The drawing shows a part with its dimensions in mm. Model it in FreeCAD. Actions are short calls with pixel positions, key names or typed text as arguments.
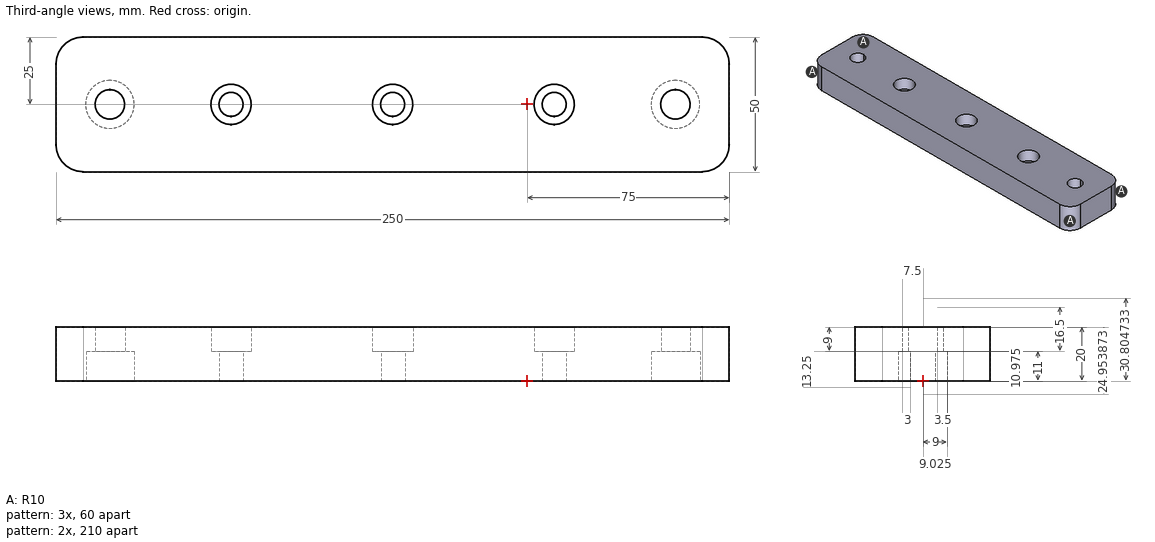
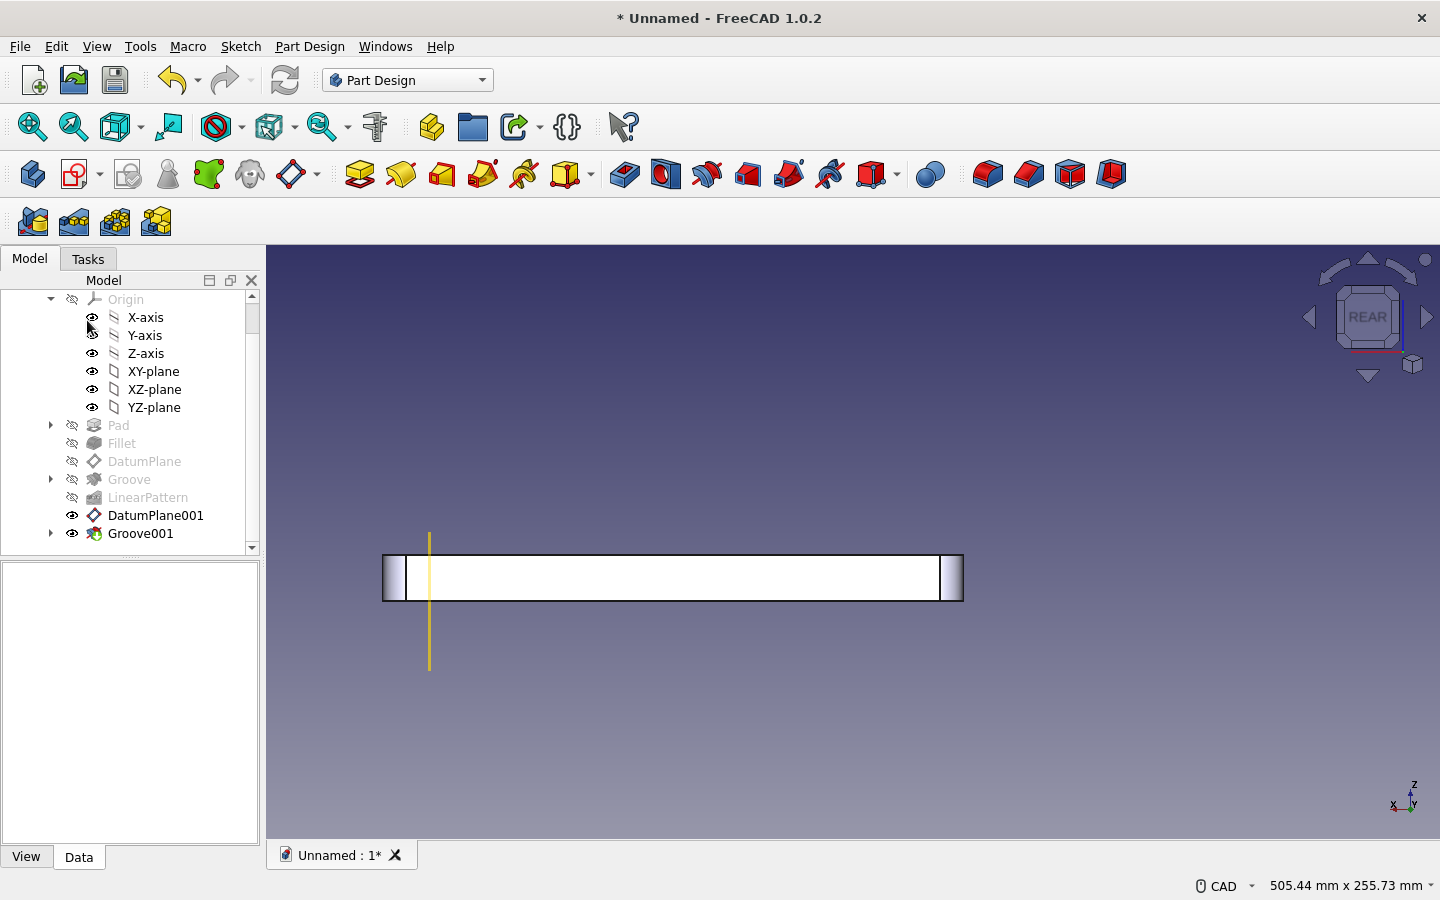
click(117, 515)
key(space)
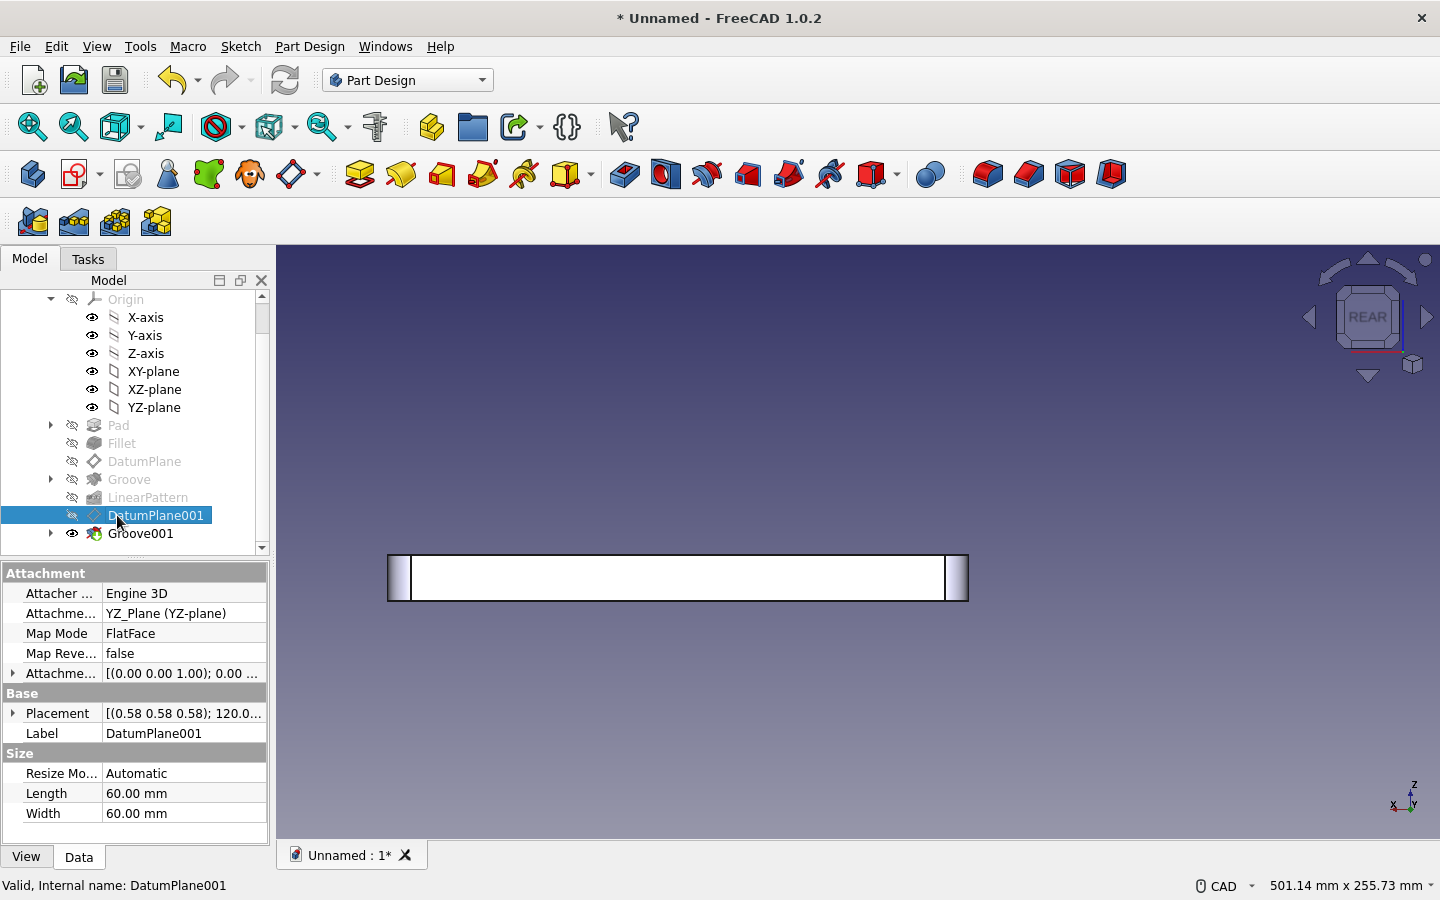
click(117, 533)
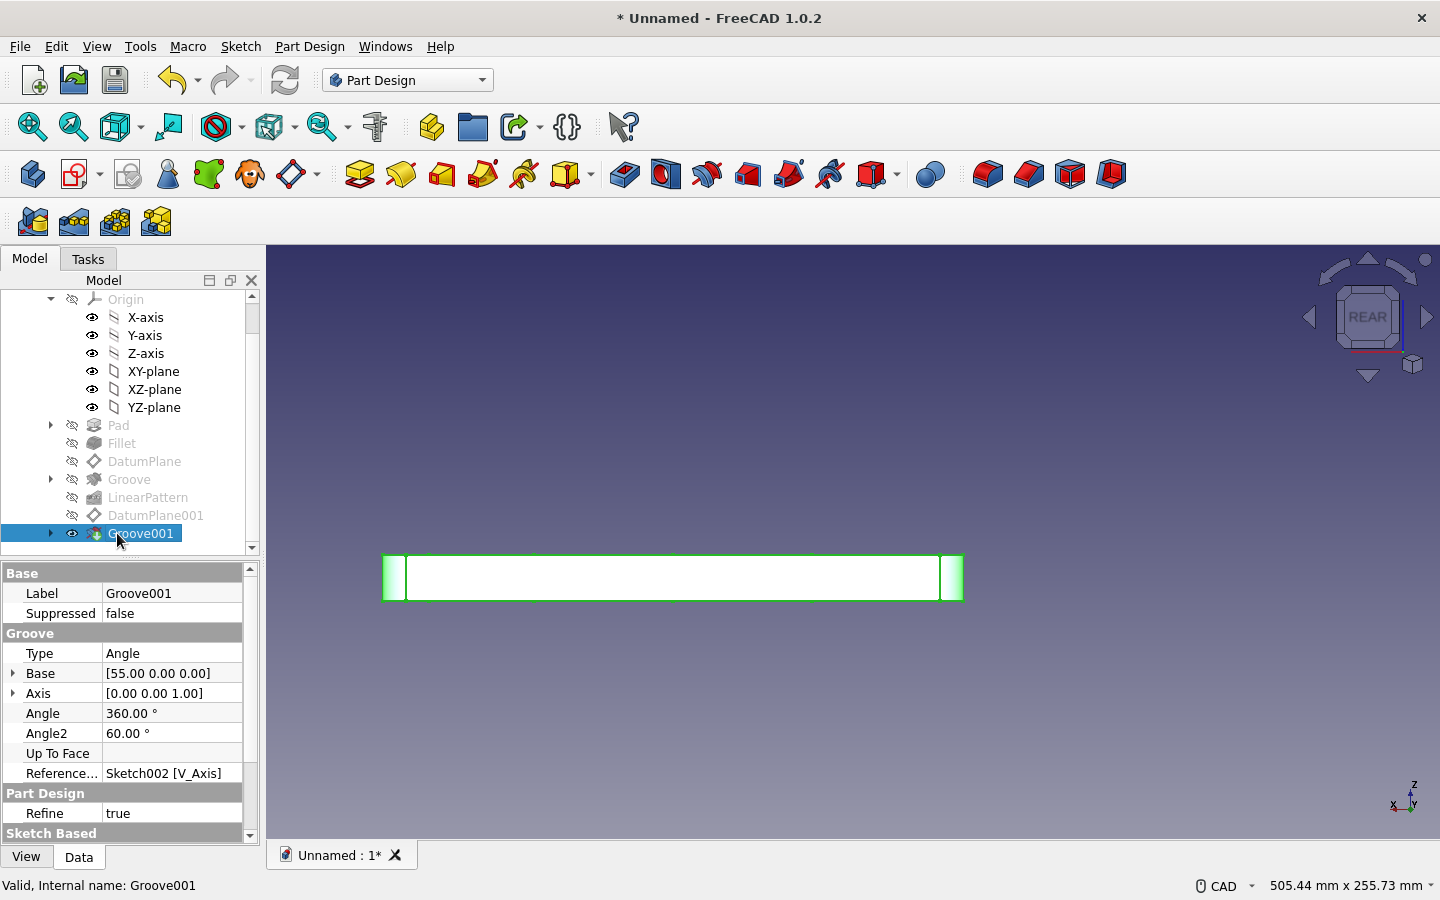
click(74, 222)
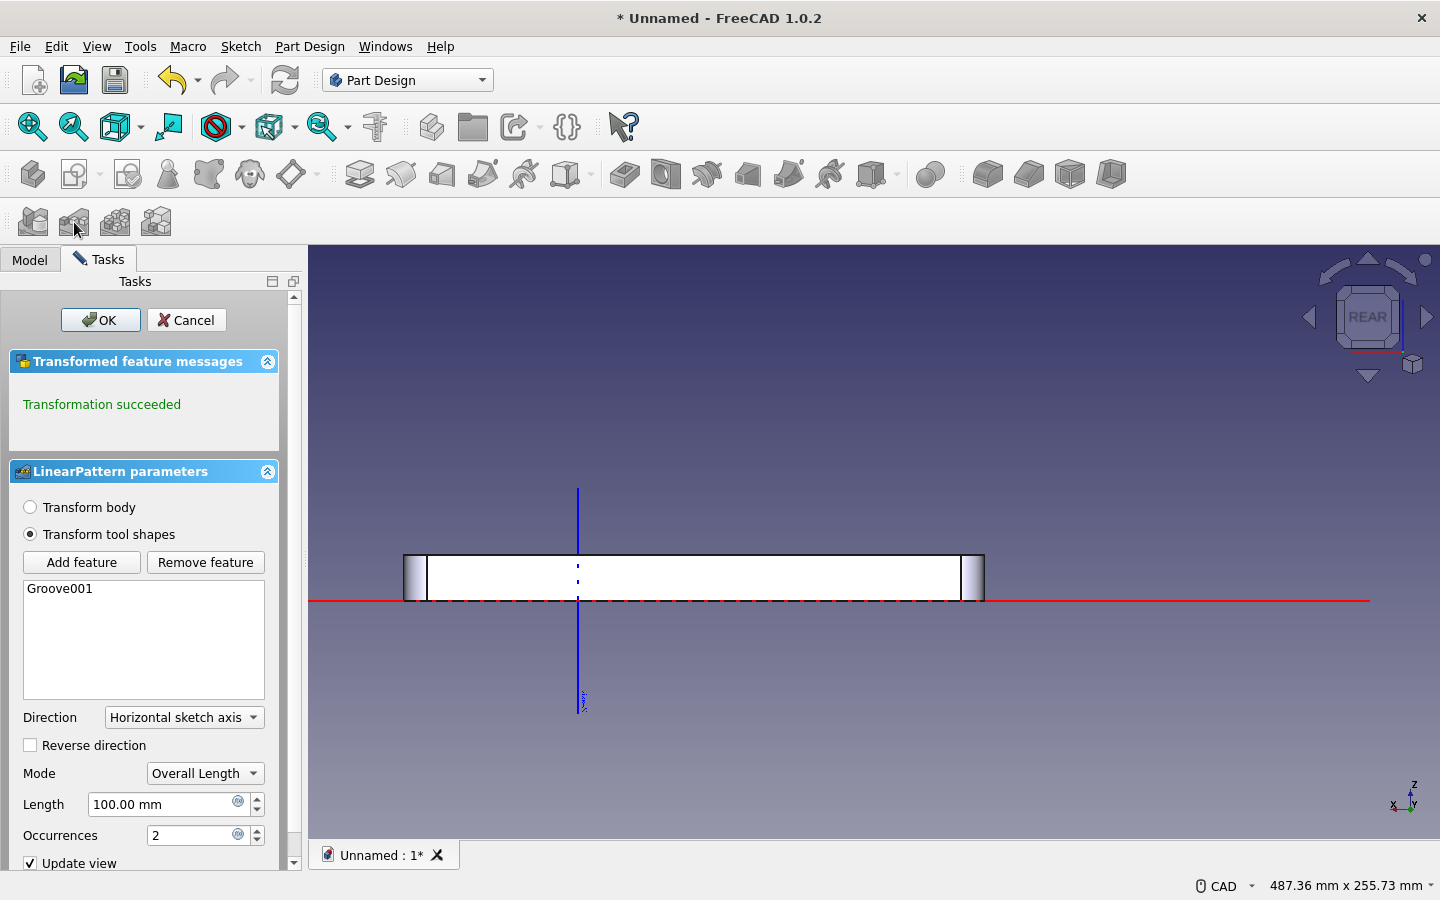
click(185, 718)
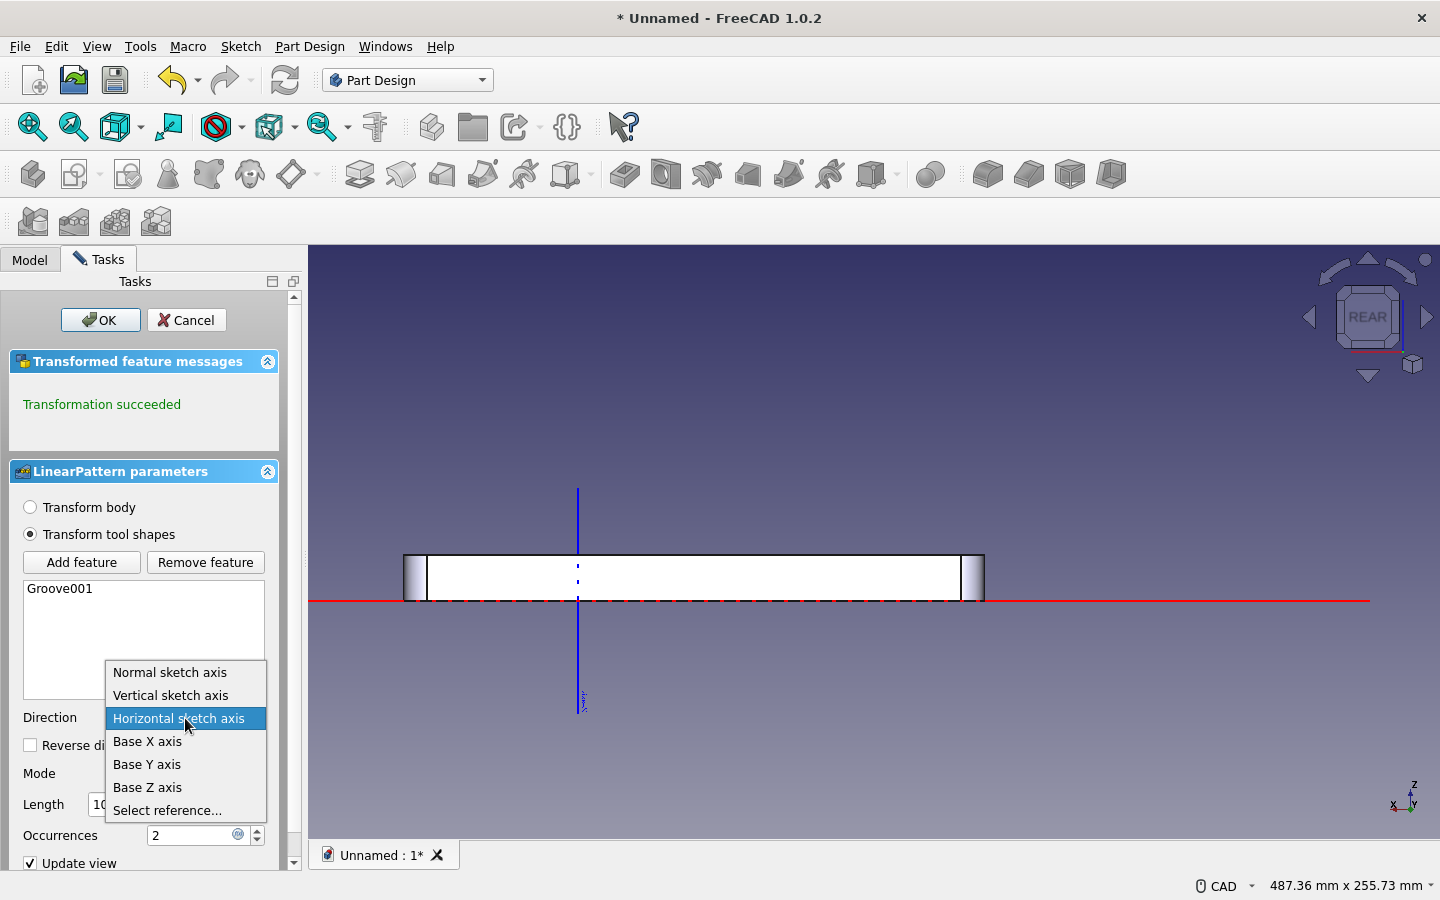
click(184, 742)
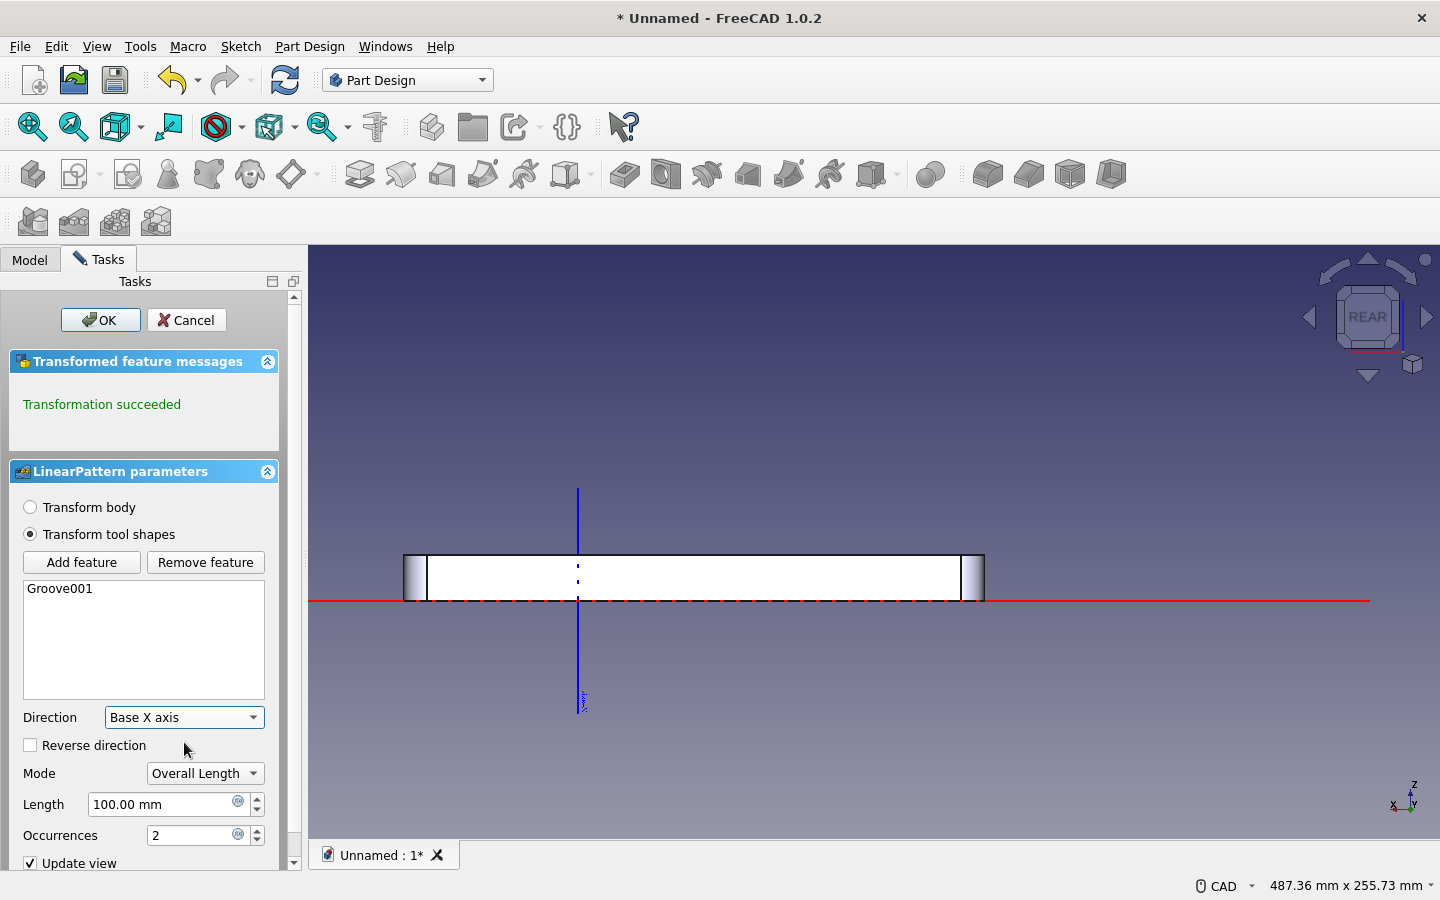
click(206, 774)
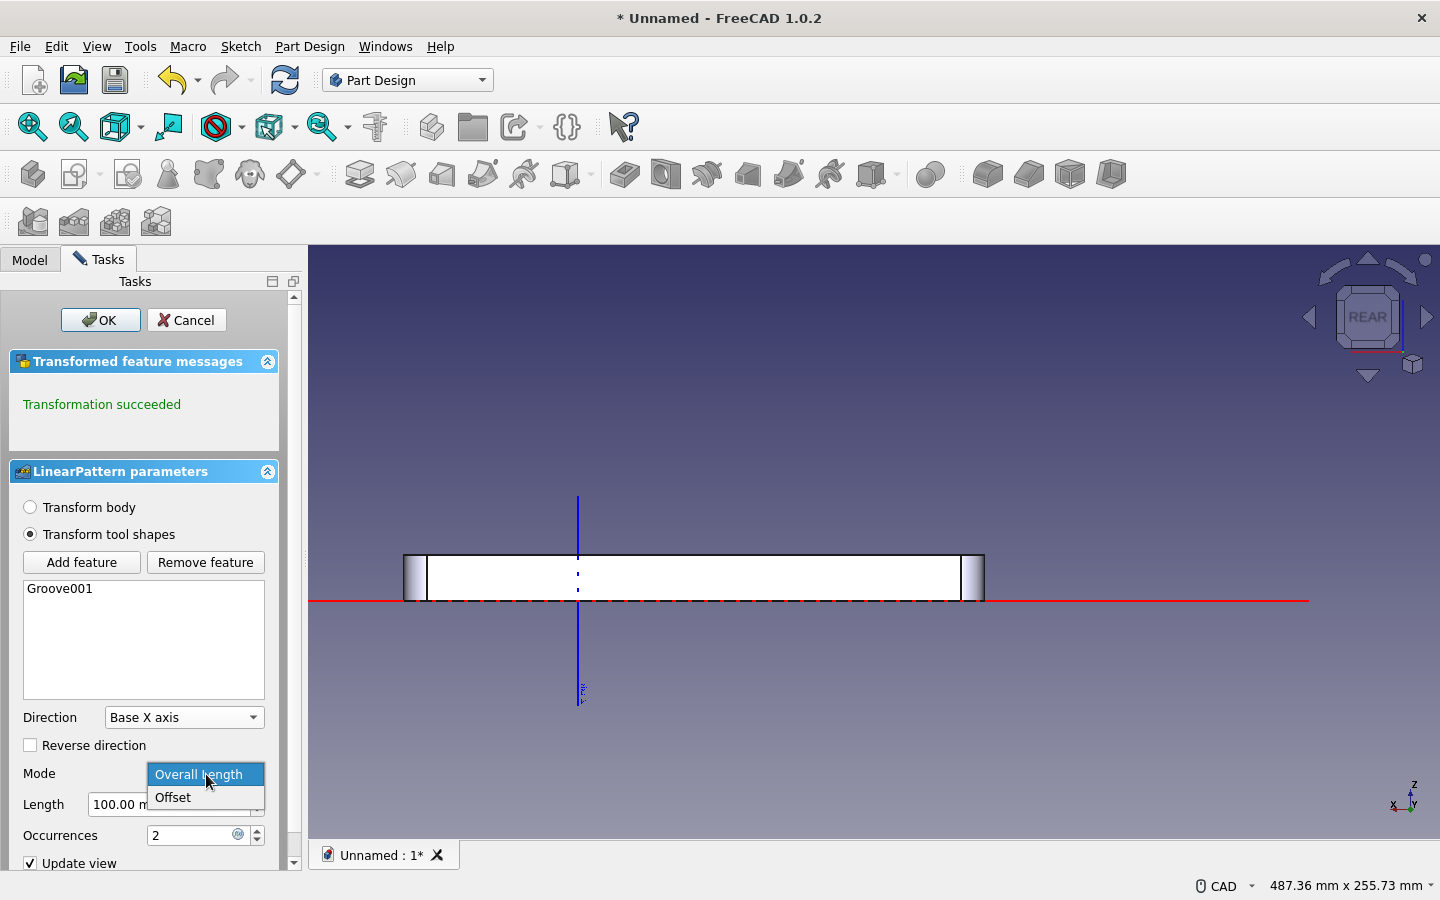
click(204, 798)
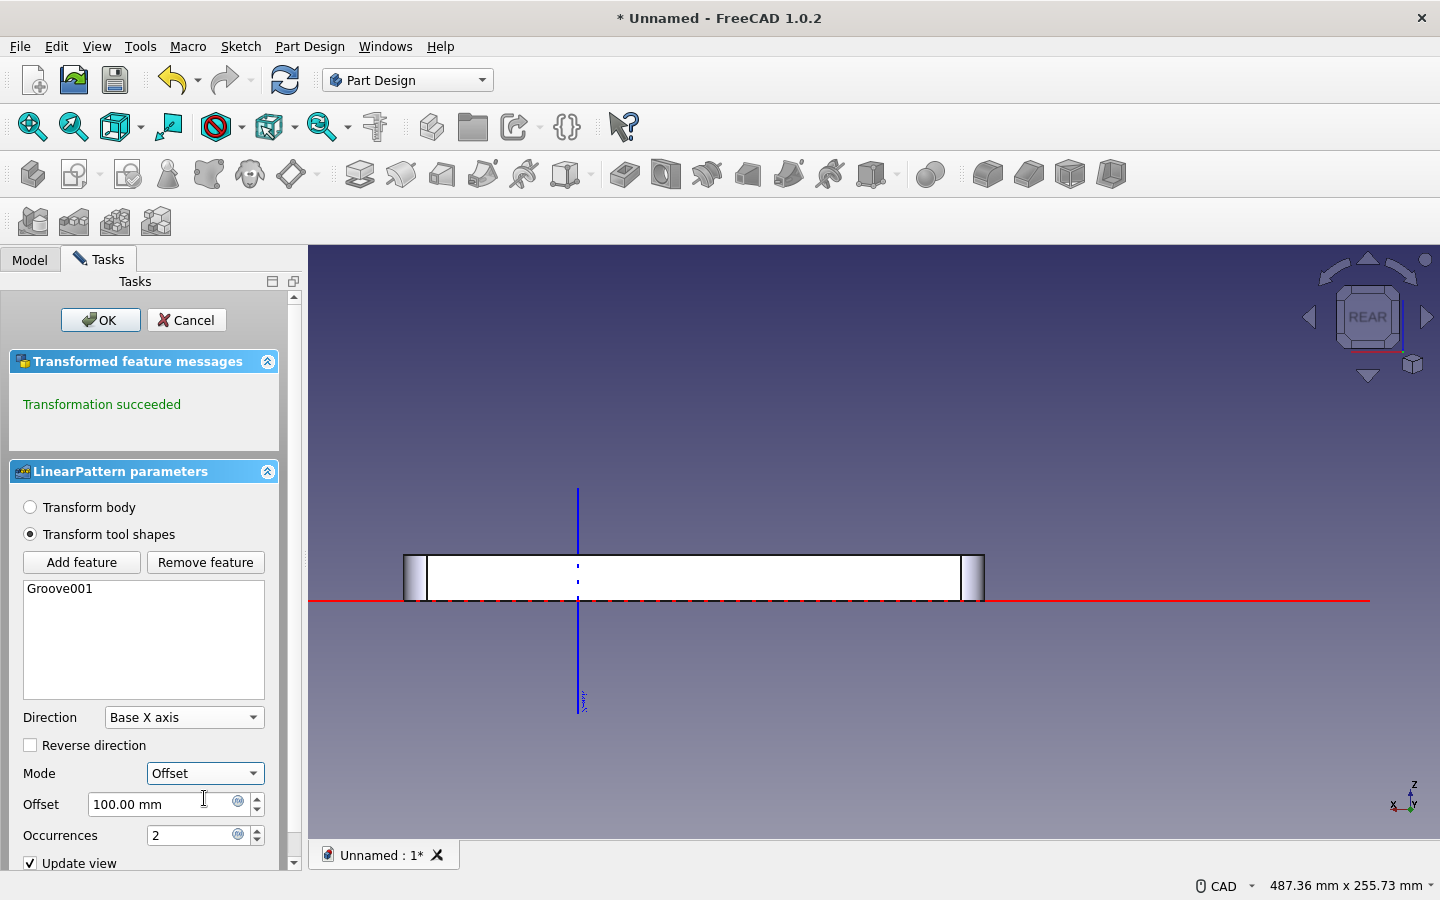
triple_click(170, 804)